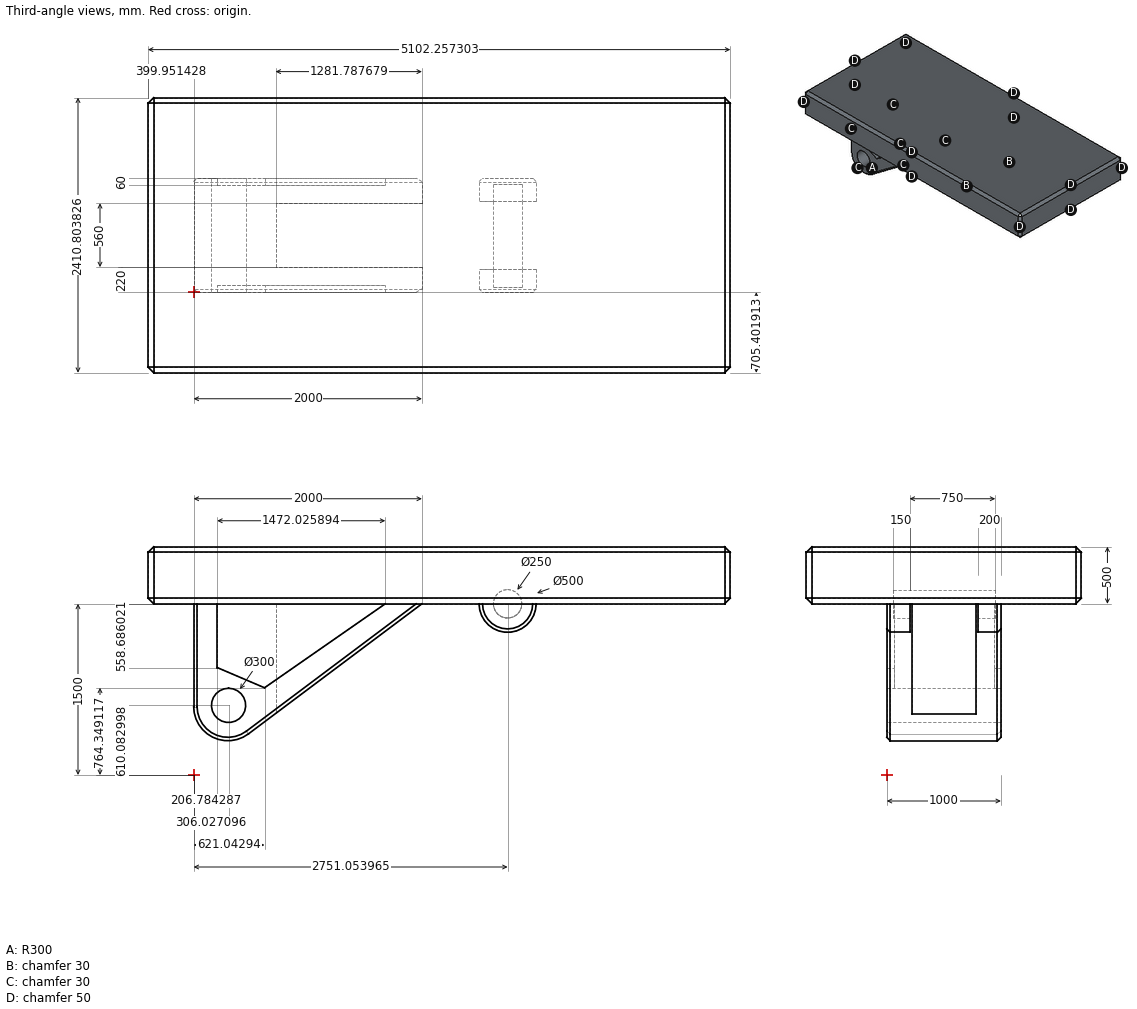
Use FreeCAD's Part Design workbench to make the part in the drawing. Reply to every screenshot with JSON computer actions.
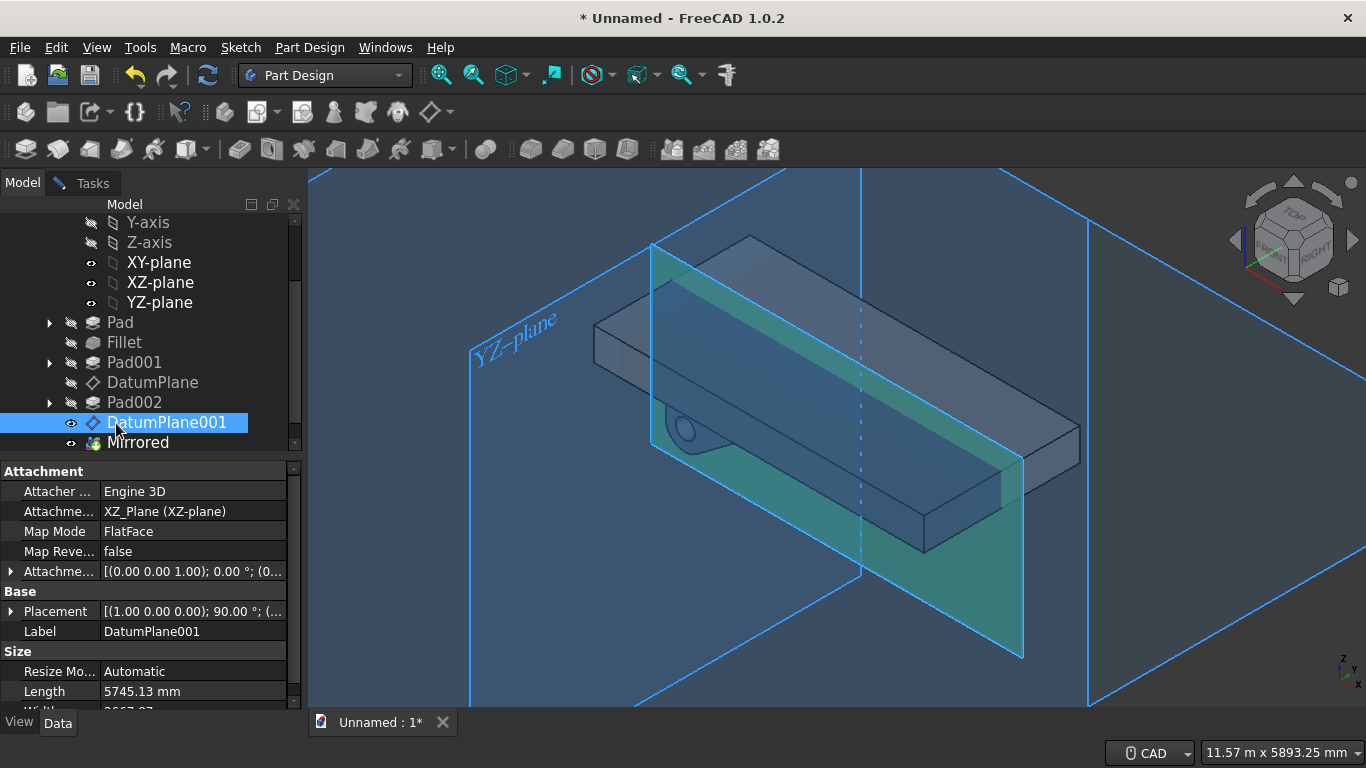
{"action": "left_click", "coordinate": [84, 182]}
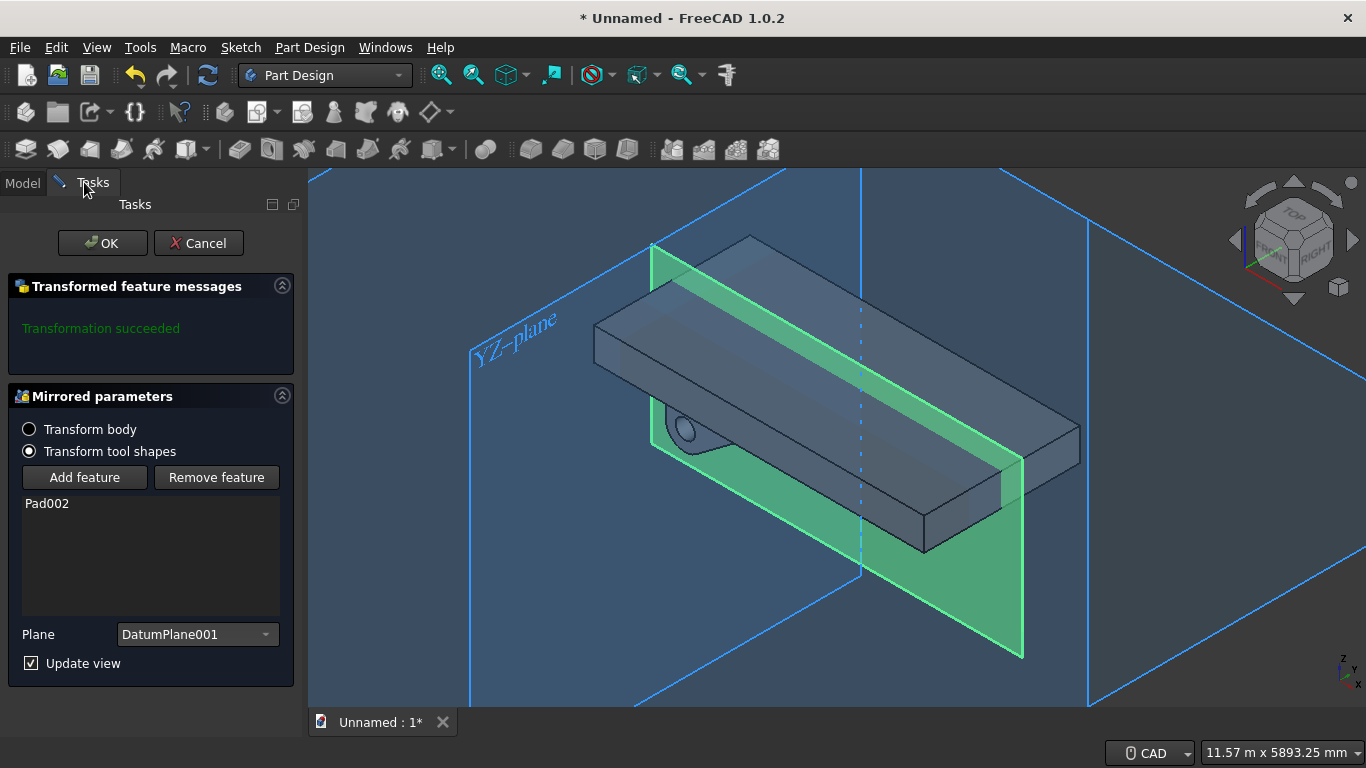
{"action": "left_click", "coordinate": [103, 243]}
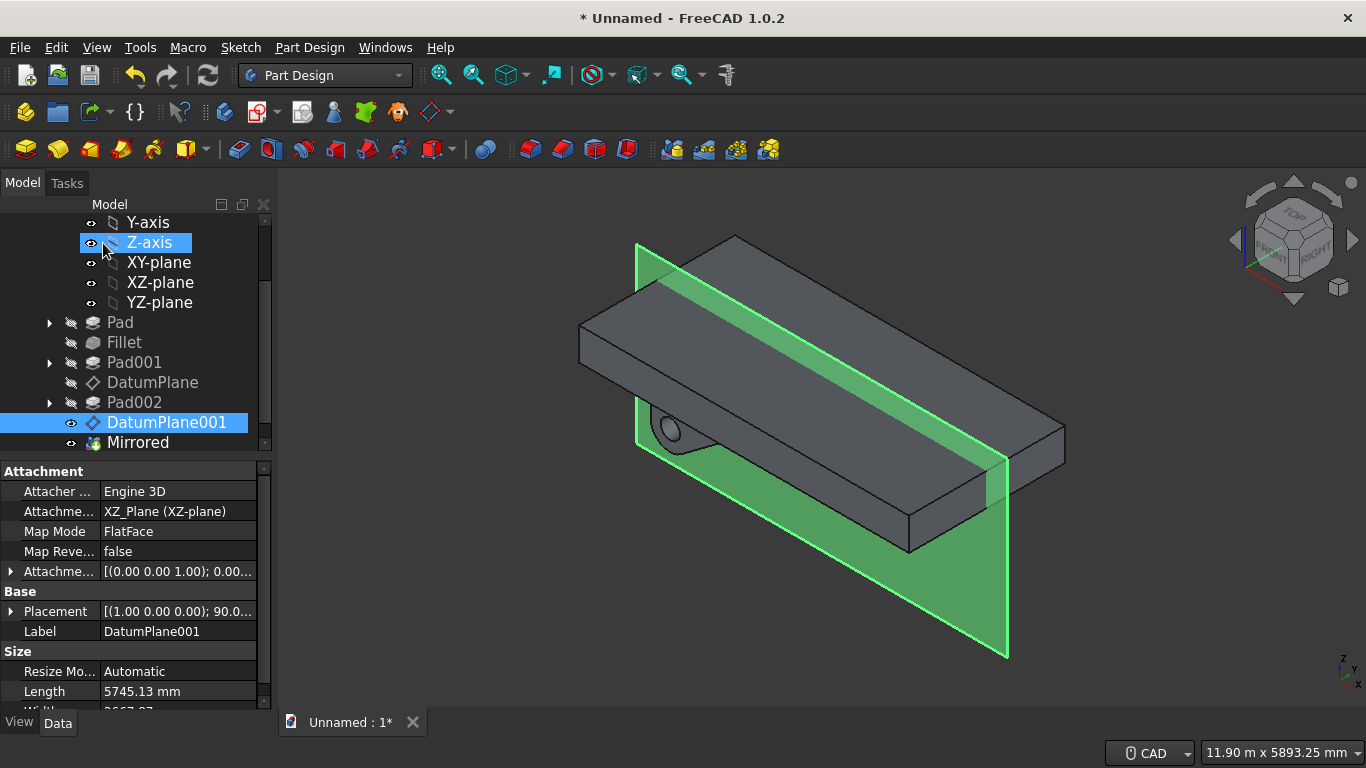
{"action": "left_click", "coordinate": [116, 423]}
{"action": "key", "text": "space"}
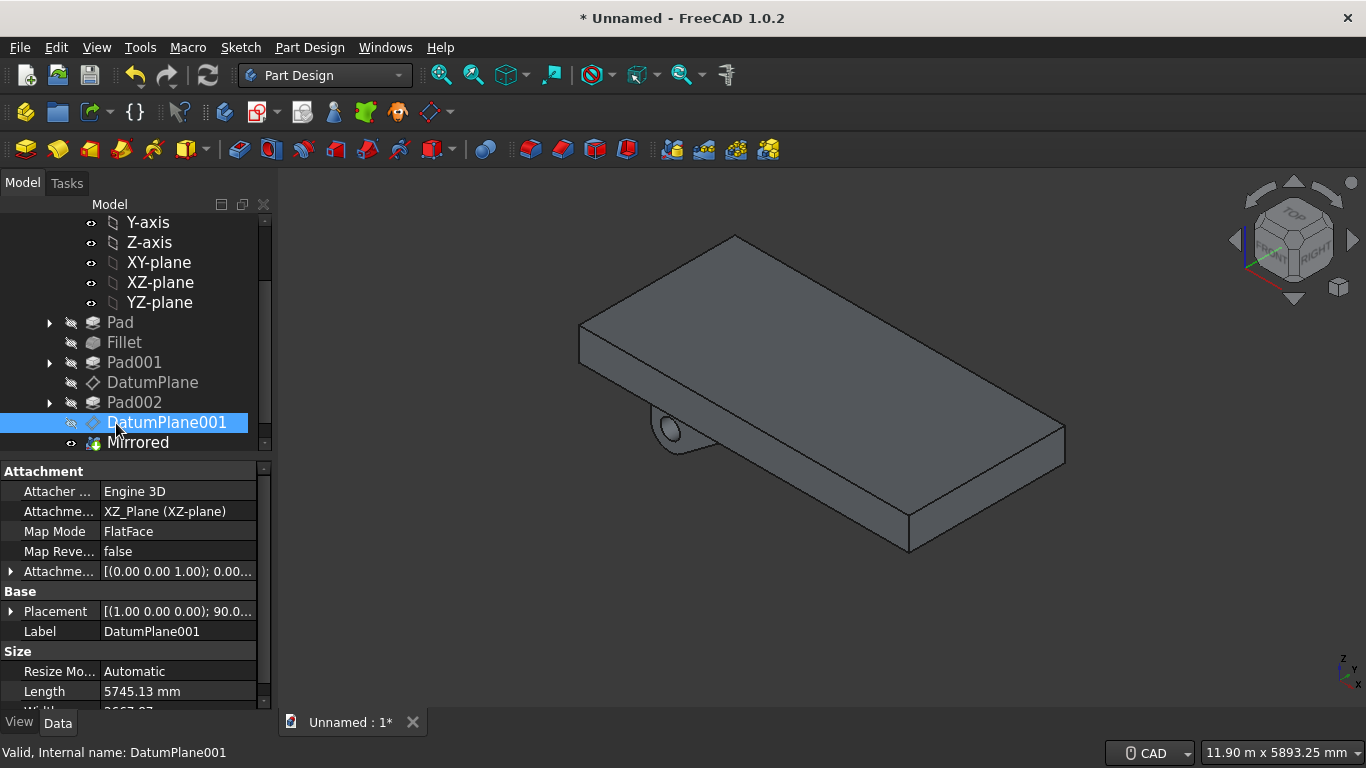
{"action": "scroll", "coordinate": [160, 338], "scroll_direction": "down", "scroll_amount": 3}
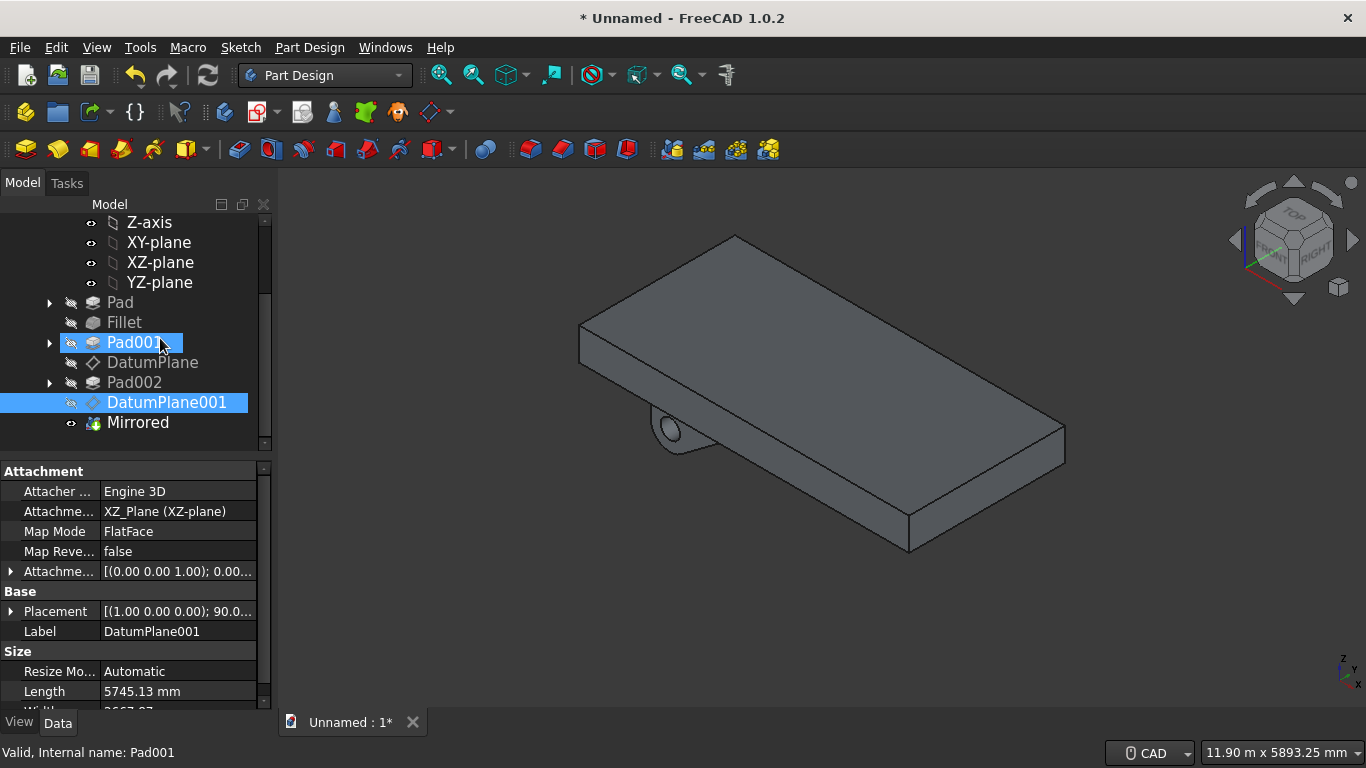
{"action": "scroll", "coordinate": [160, 318], "scroll_direction": "up", "scroll_amount": 15}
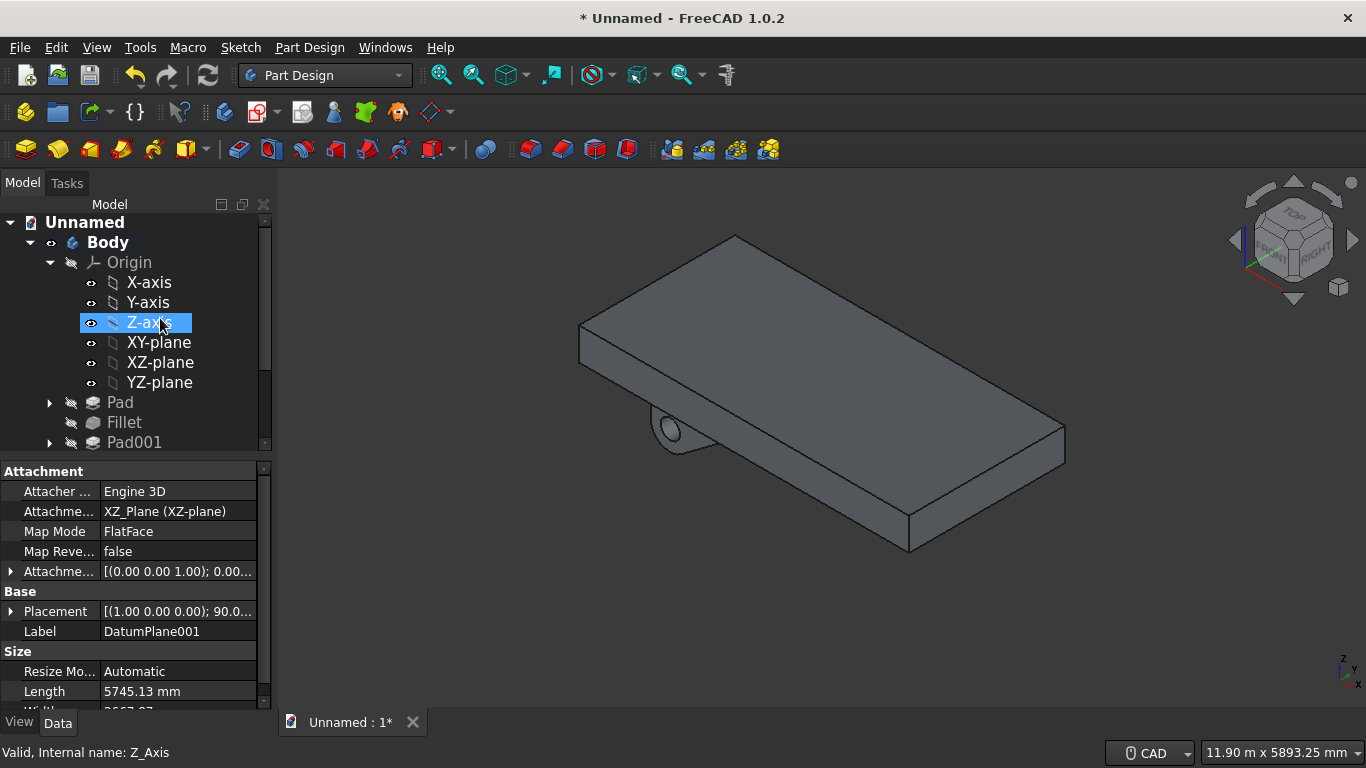
{"action": "left_click", "coordinate": [136, 363]}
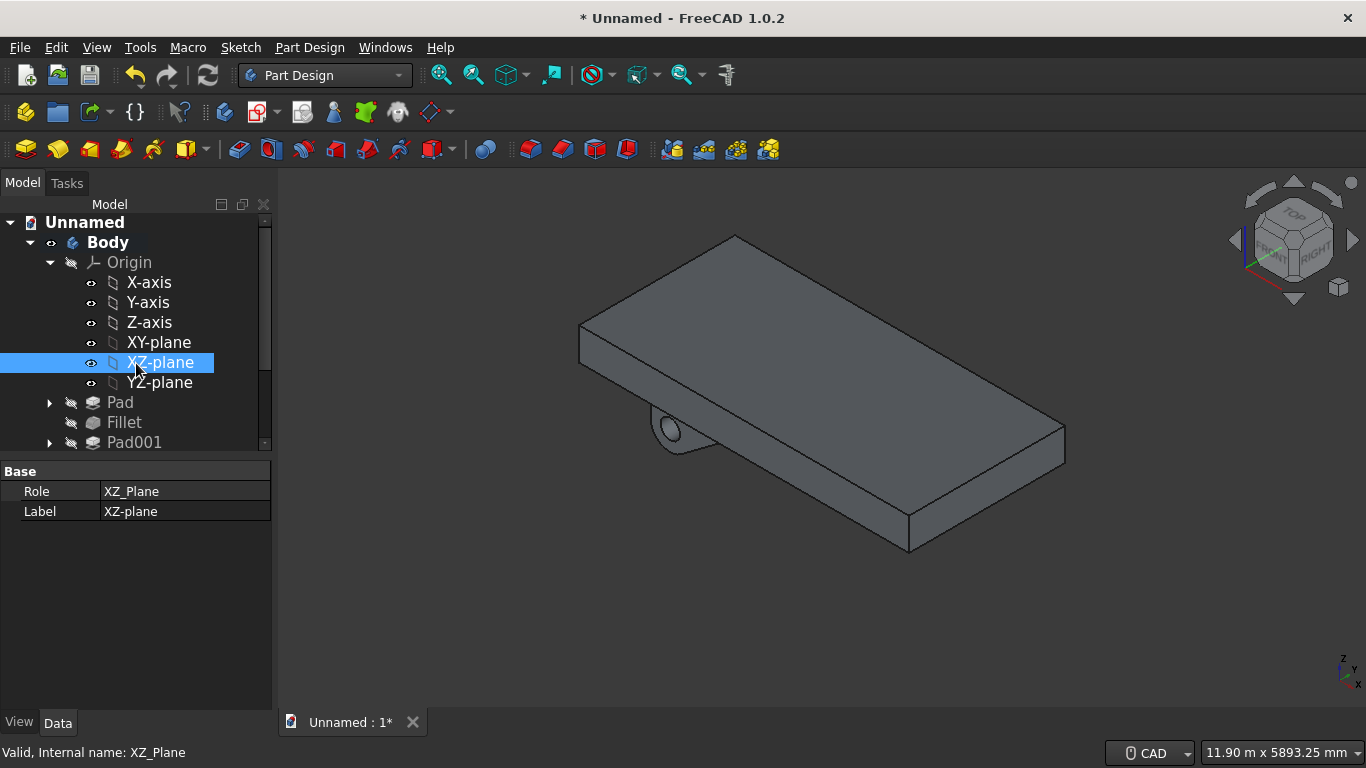
{"action": "left_click", "coordinate": [430, 112]}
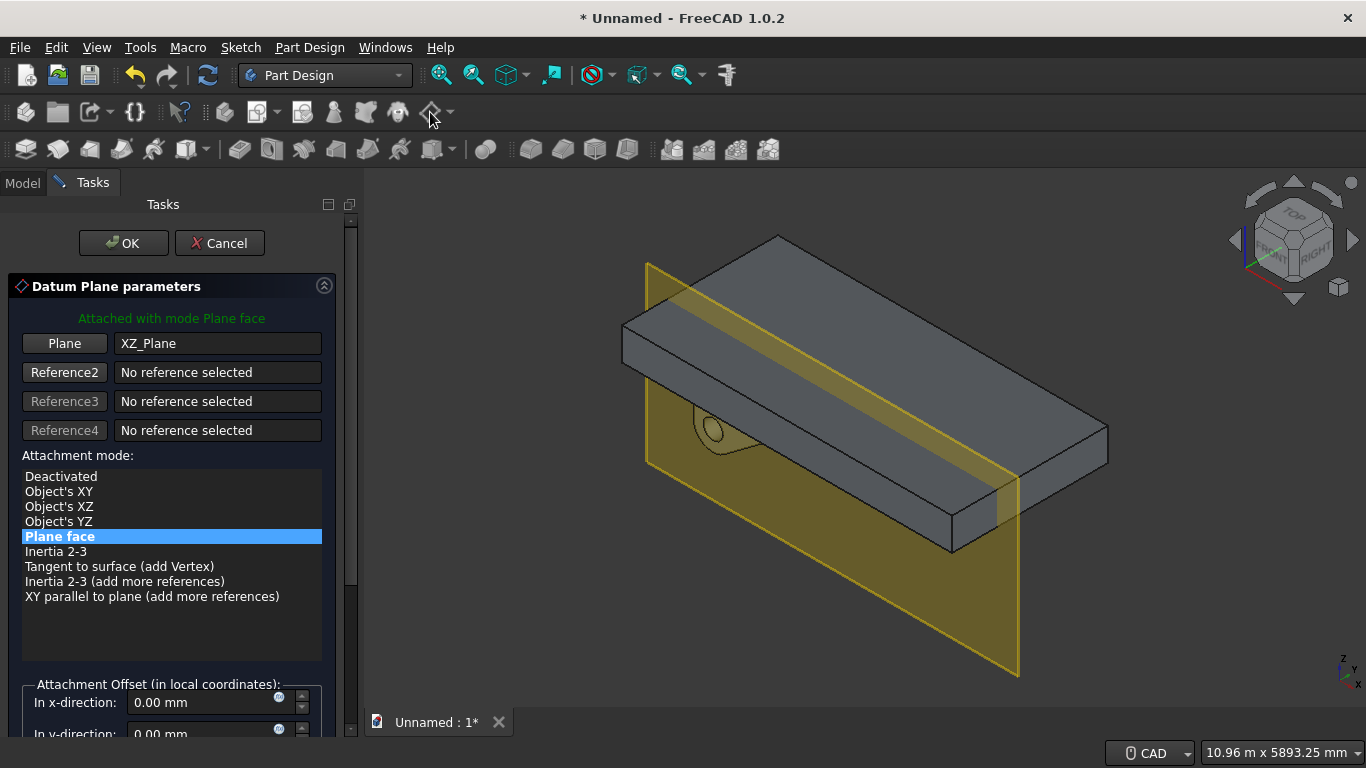
{"action": "scroll", "coordinate": [351, 475], "scroll_direction": "down", "scroll_amount": 2}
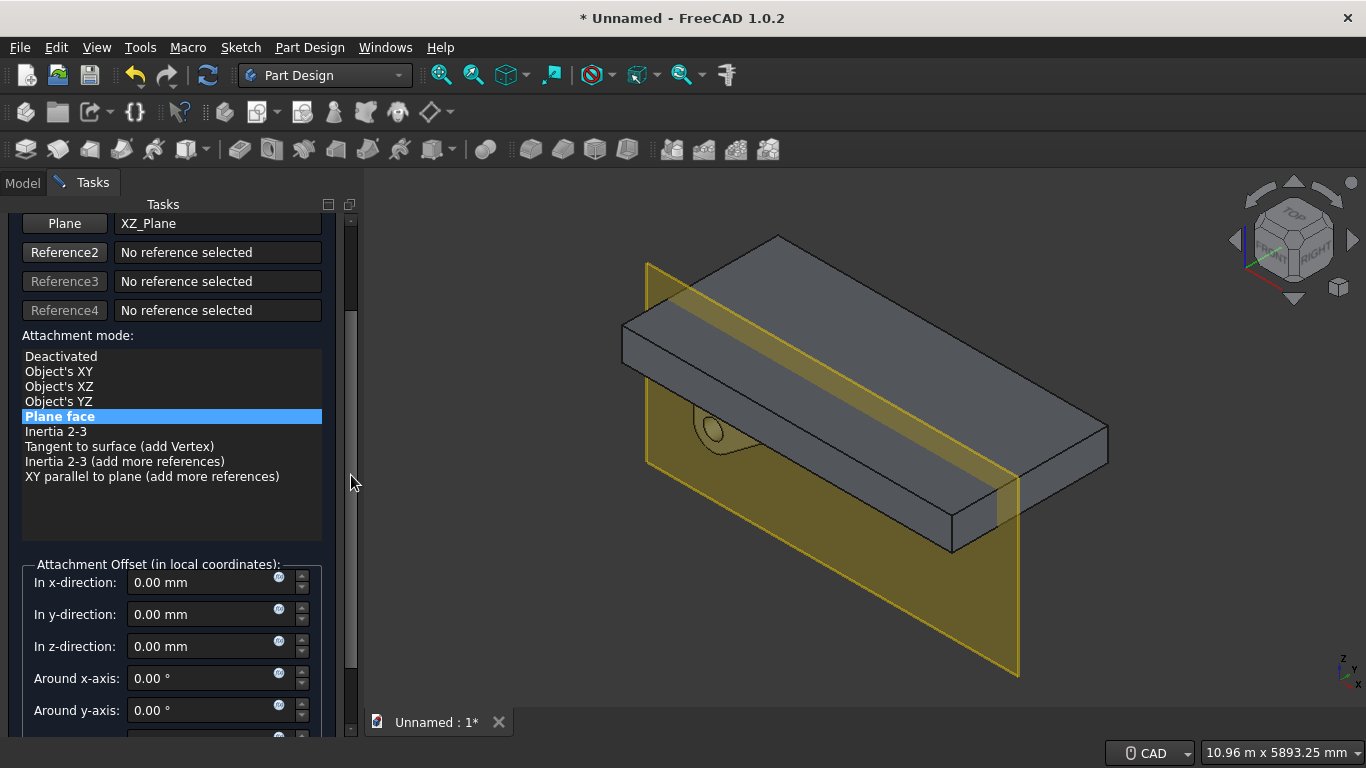
{"action": "triple_click", "coordinate": [210, 646]}